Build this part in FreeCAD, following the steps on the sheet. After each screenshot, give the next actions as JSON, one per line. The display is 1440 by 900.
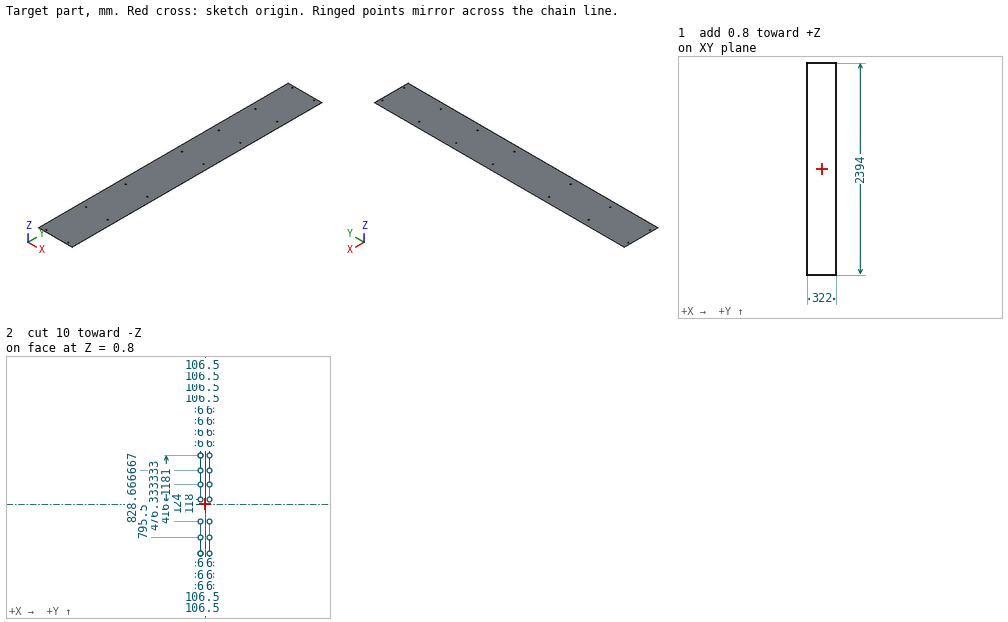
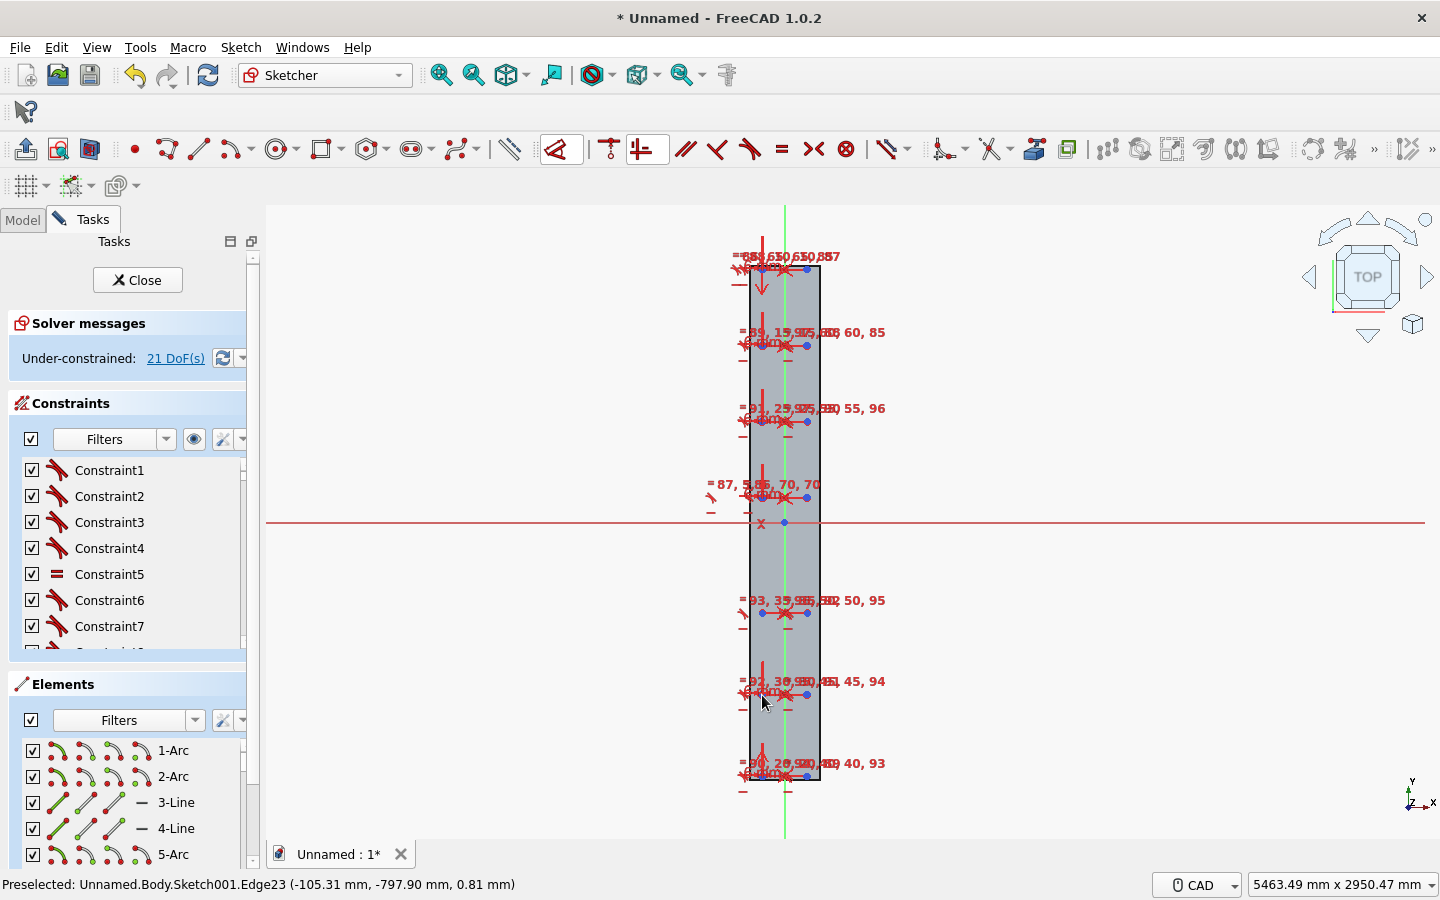
{"action": "scroll", "coordinate": [763, 613], "scroll_direction": "up", "scroll_amount": 18}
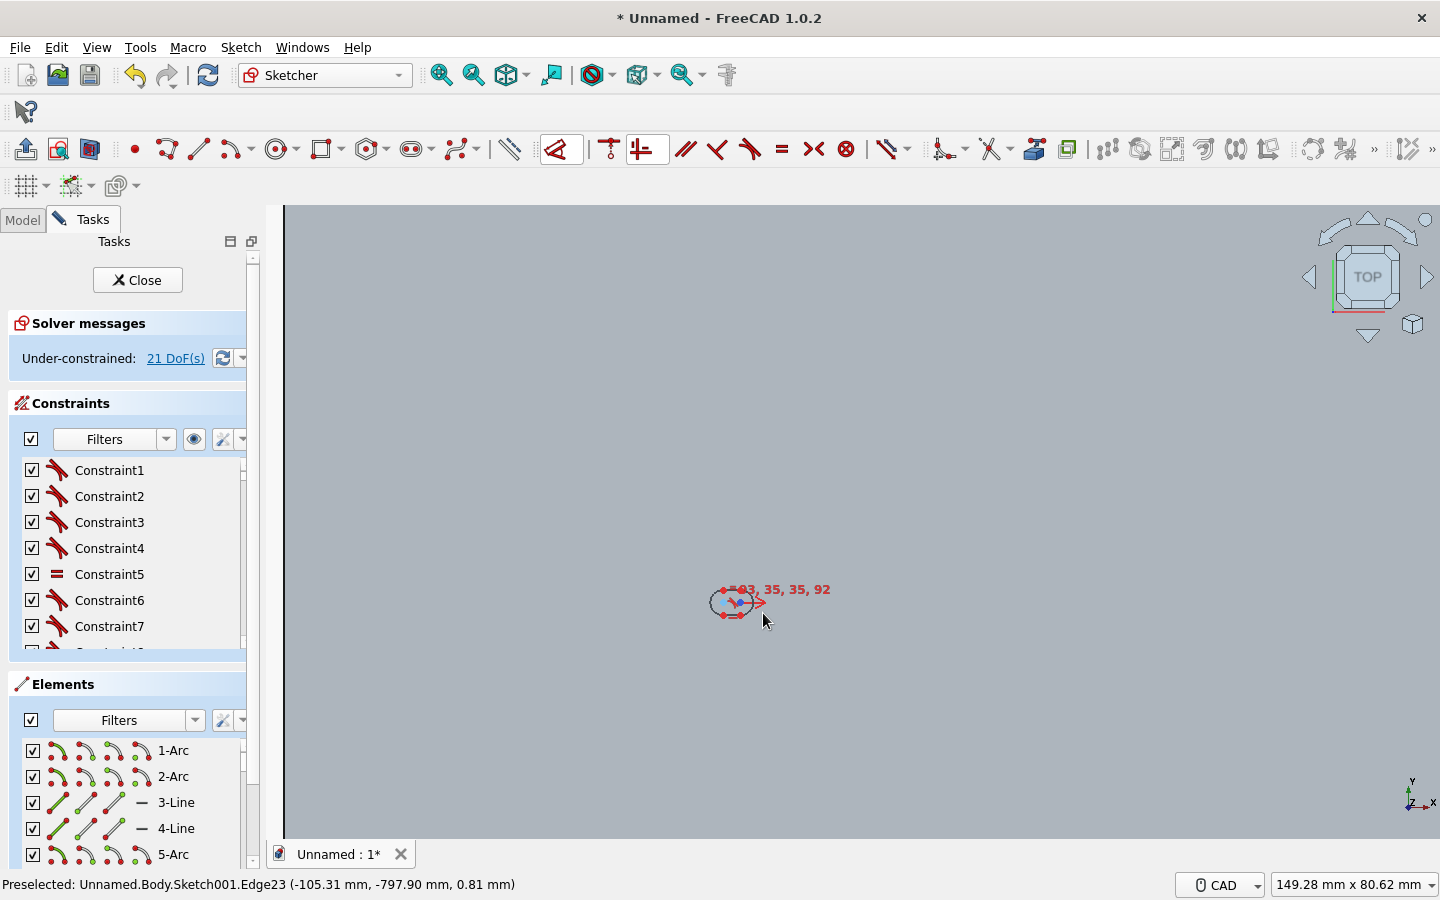
{"action": "scroll", "coordinate": [732, 590], "scroll_direction": "up", "scroll_amount": 4}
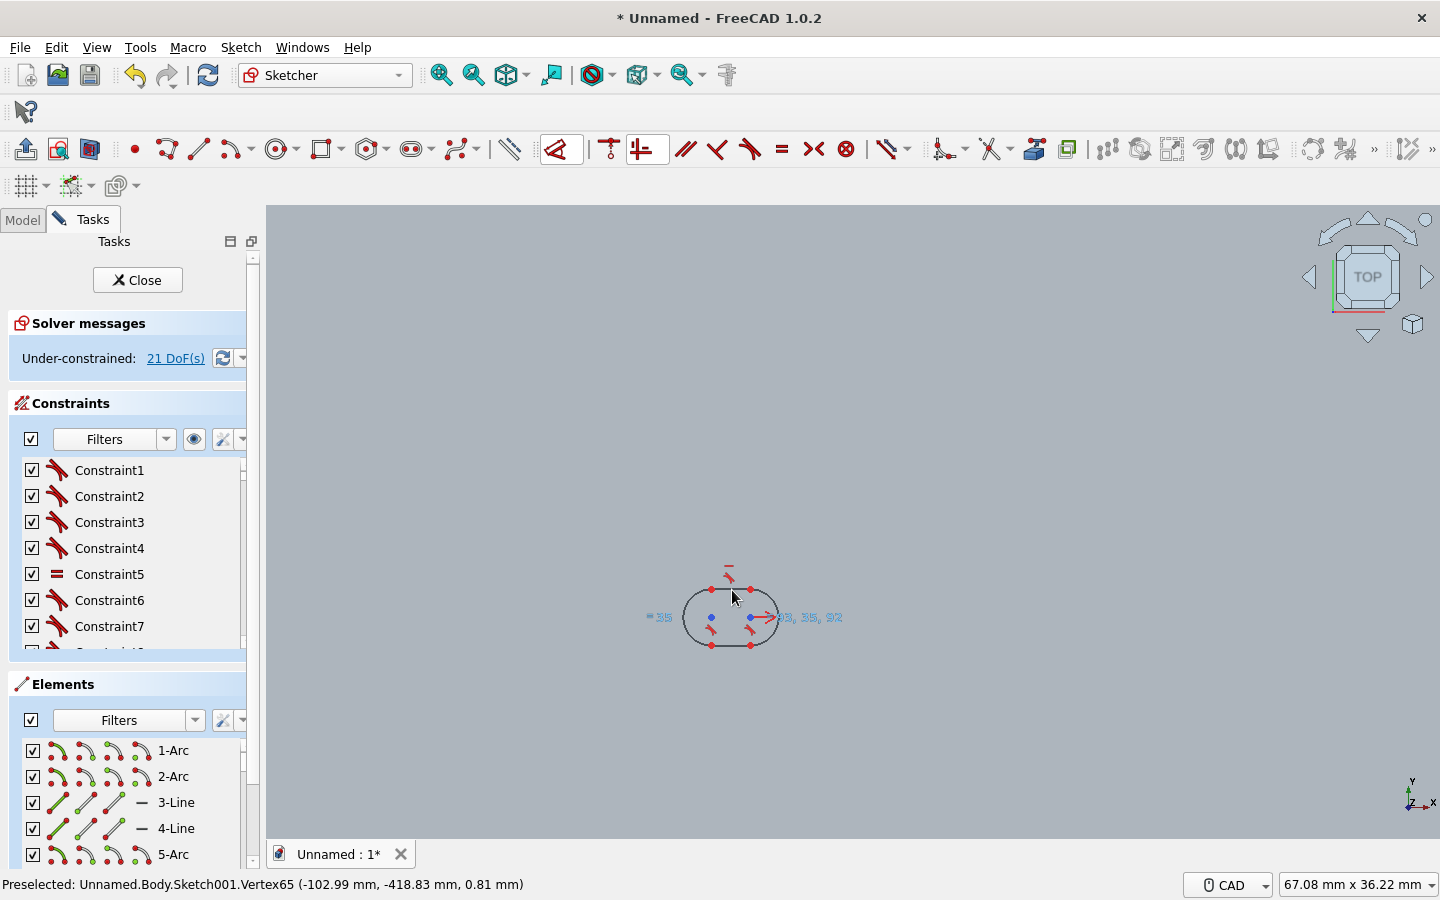
{"action": "left_click", "coordinate": [731, 589]}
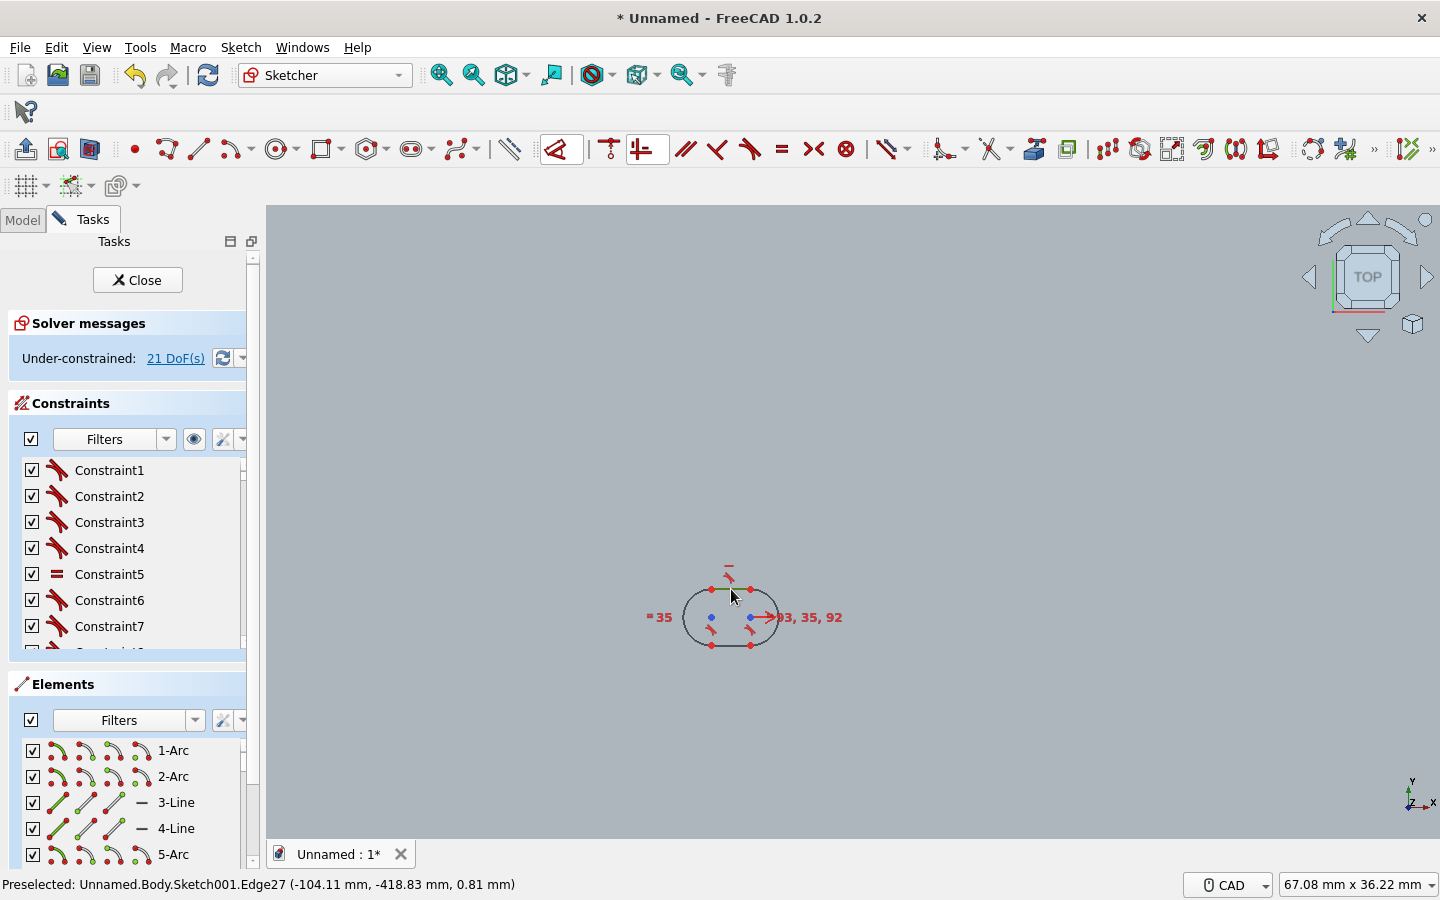
{"action": "key", "text": "l"}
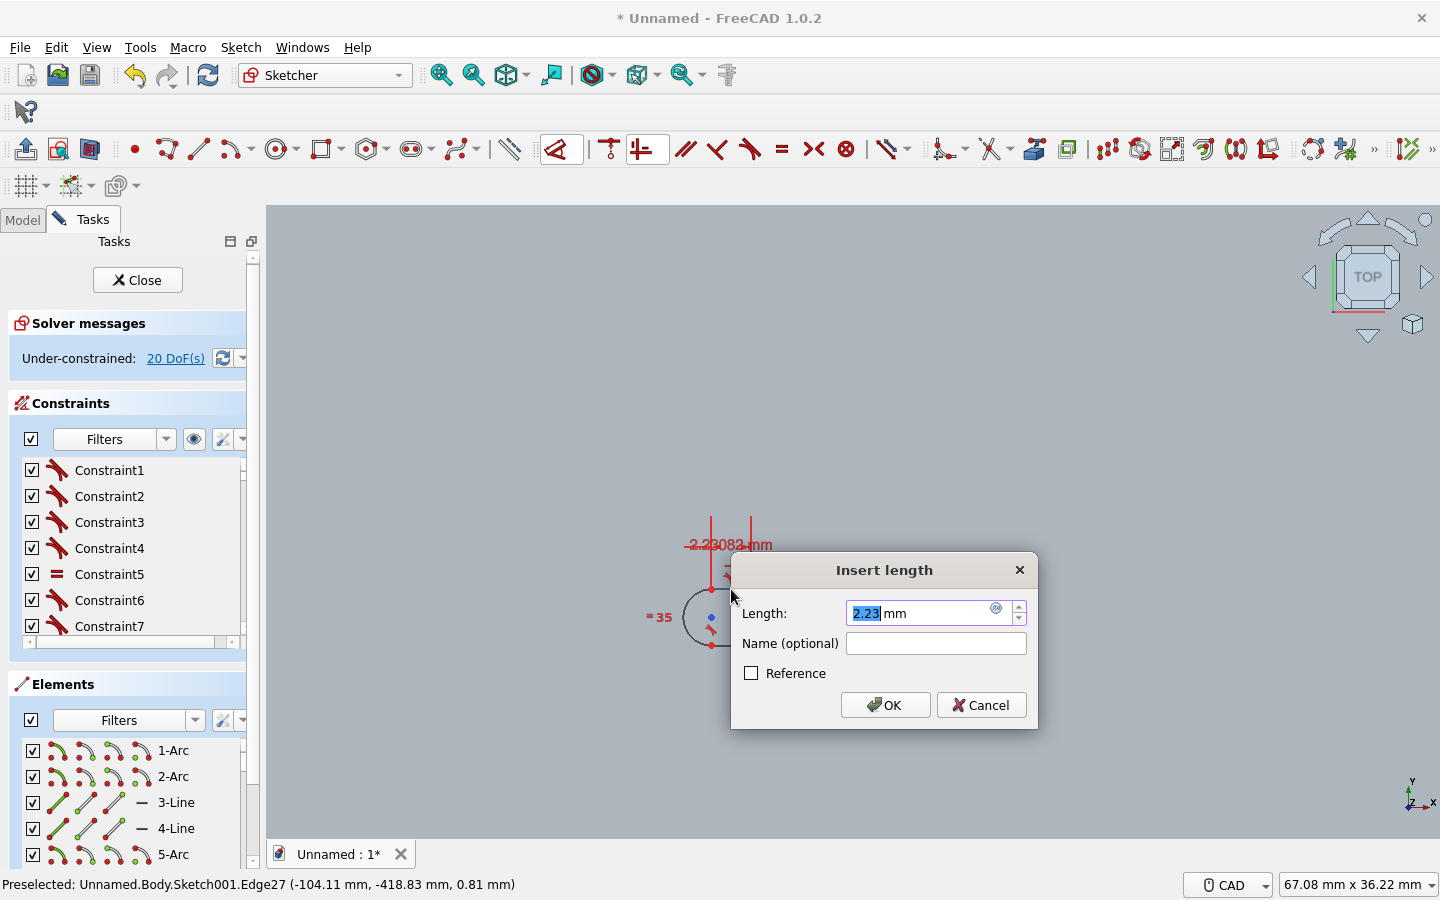
{"action": "type", "text": "6"}
{"action": "key", "text": "Return"}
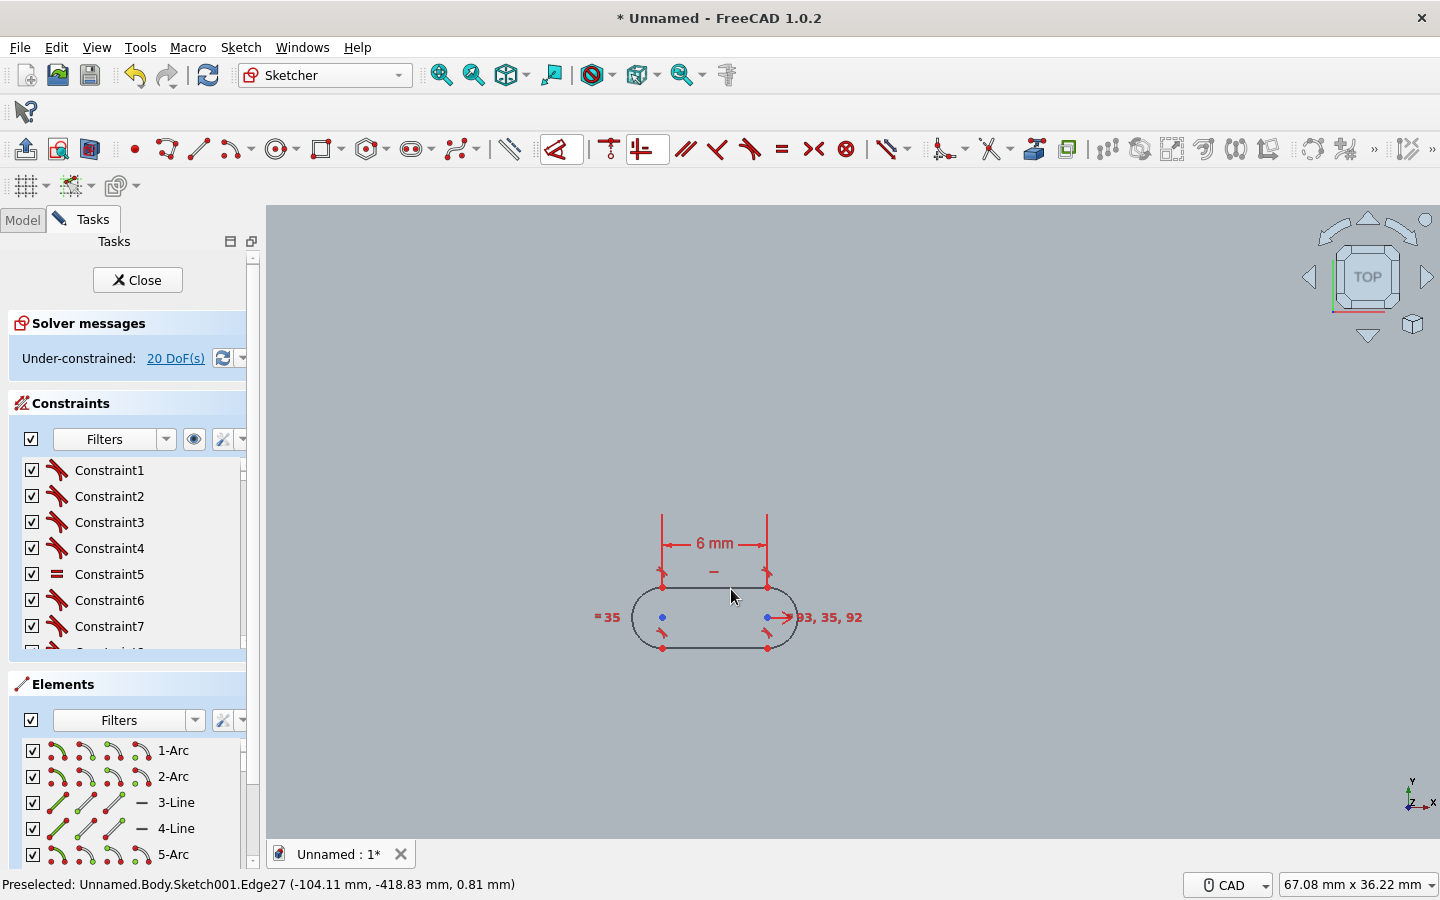
{"action": "scroll", "coordinate": [784, 522], "scroll_direction": "down", "scroll_amount": 15}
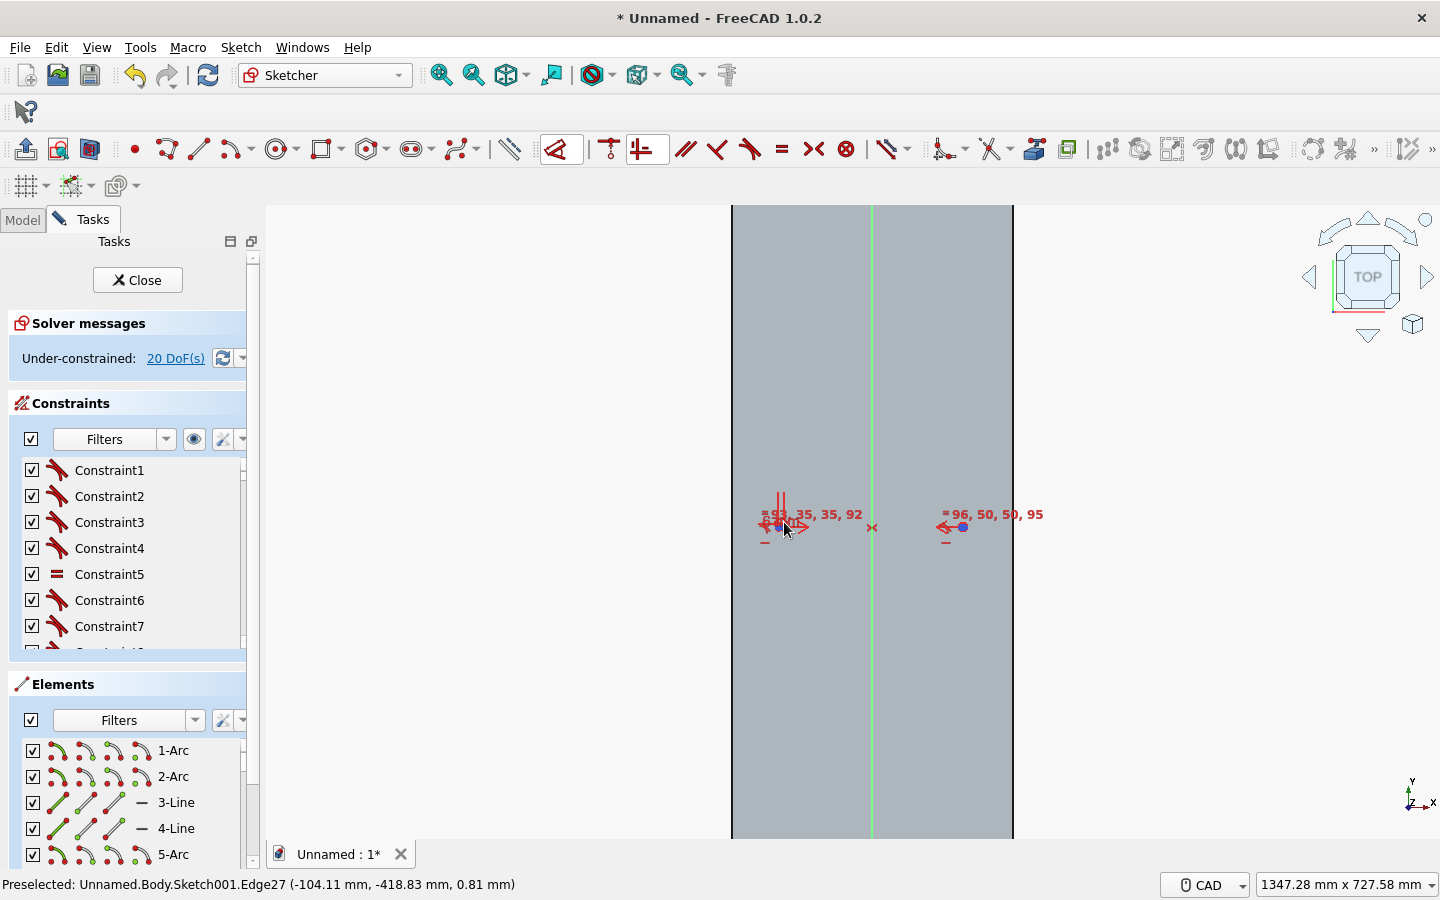
{"action": "scroll", "coordinate": [762, 613], "scroll_direction": "down", "scroll_amount": 8}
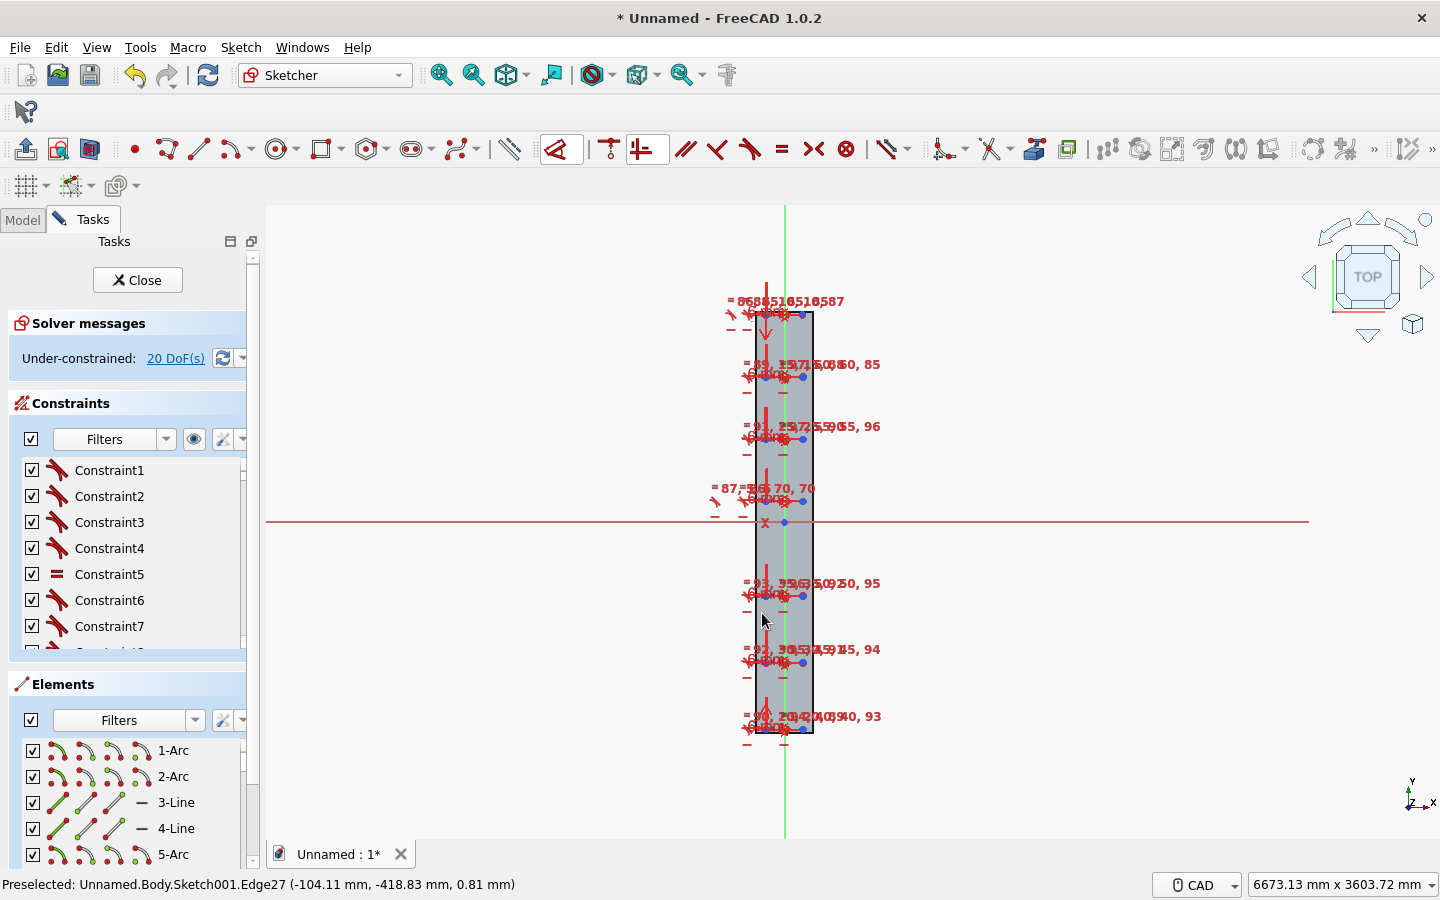
{"action": "scroll", "coordinate": [803, 729], "scroll_direction": "up", "scroll_amount": 19}